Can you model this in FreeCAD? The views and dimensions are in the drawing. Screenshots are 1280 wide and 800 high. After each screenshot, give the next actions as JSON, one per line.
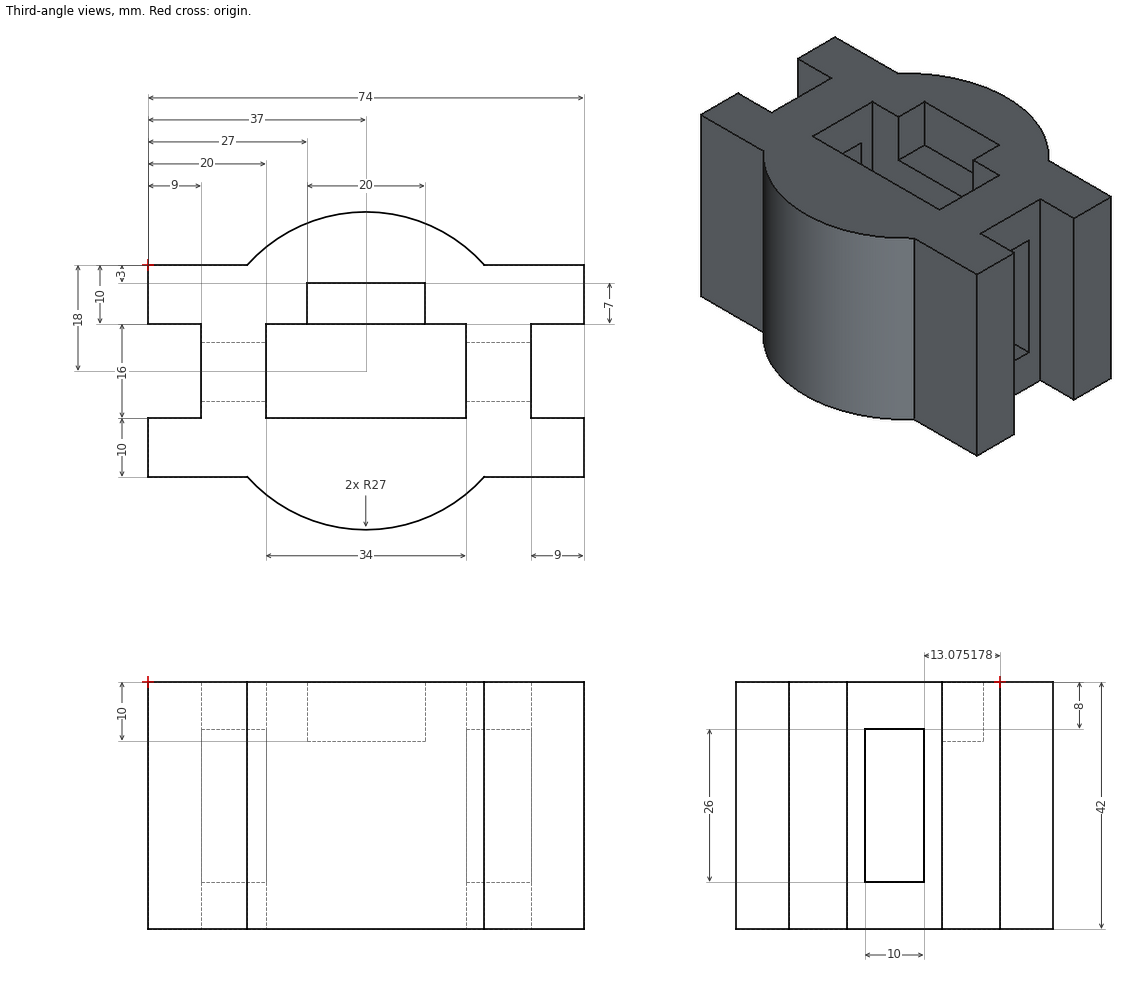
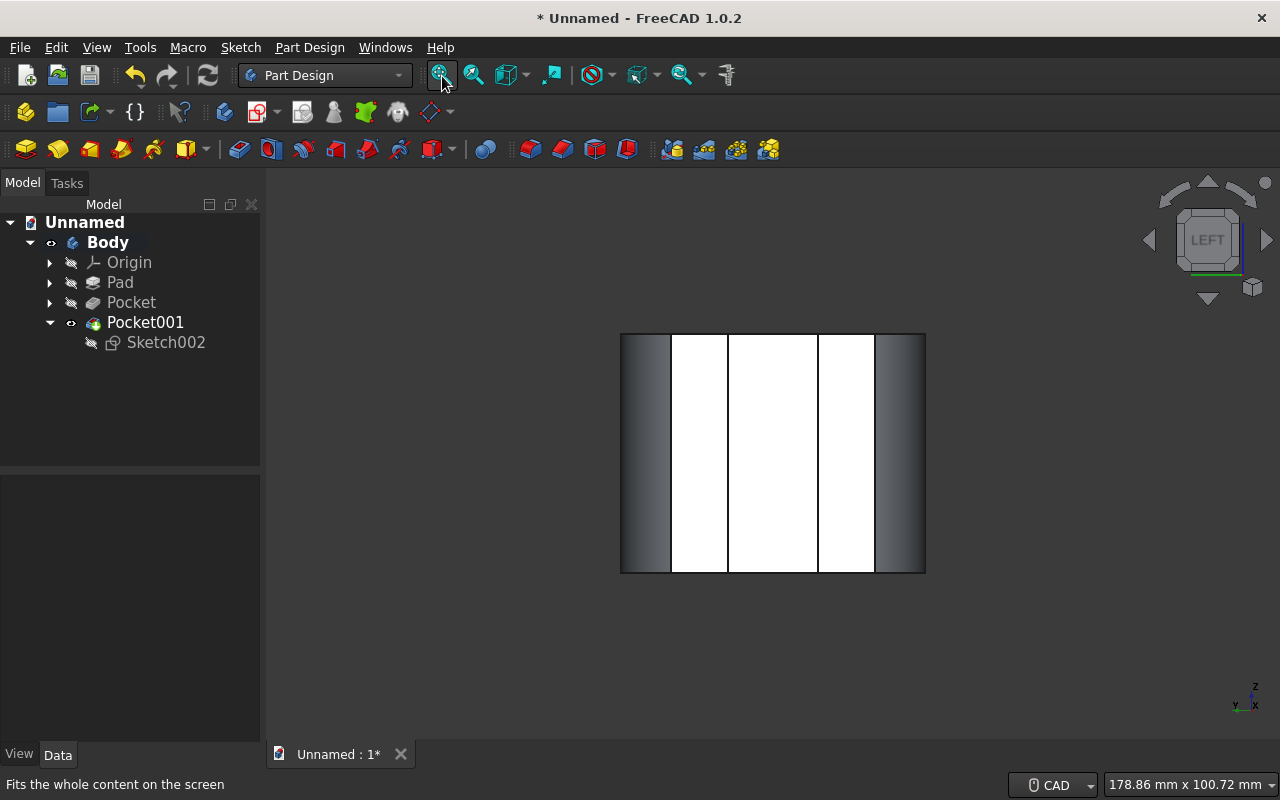
{"action": "left_click", "coordinate": [773, 384]}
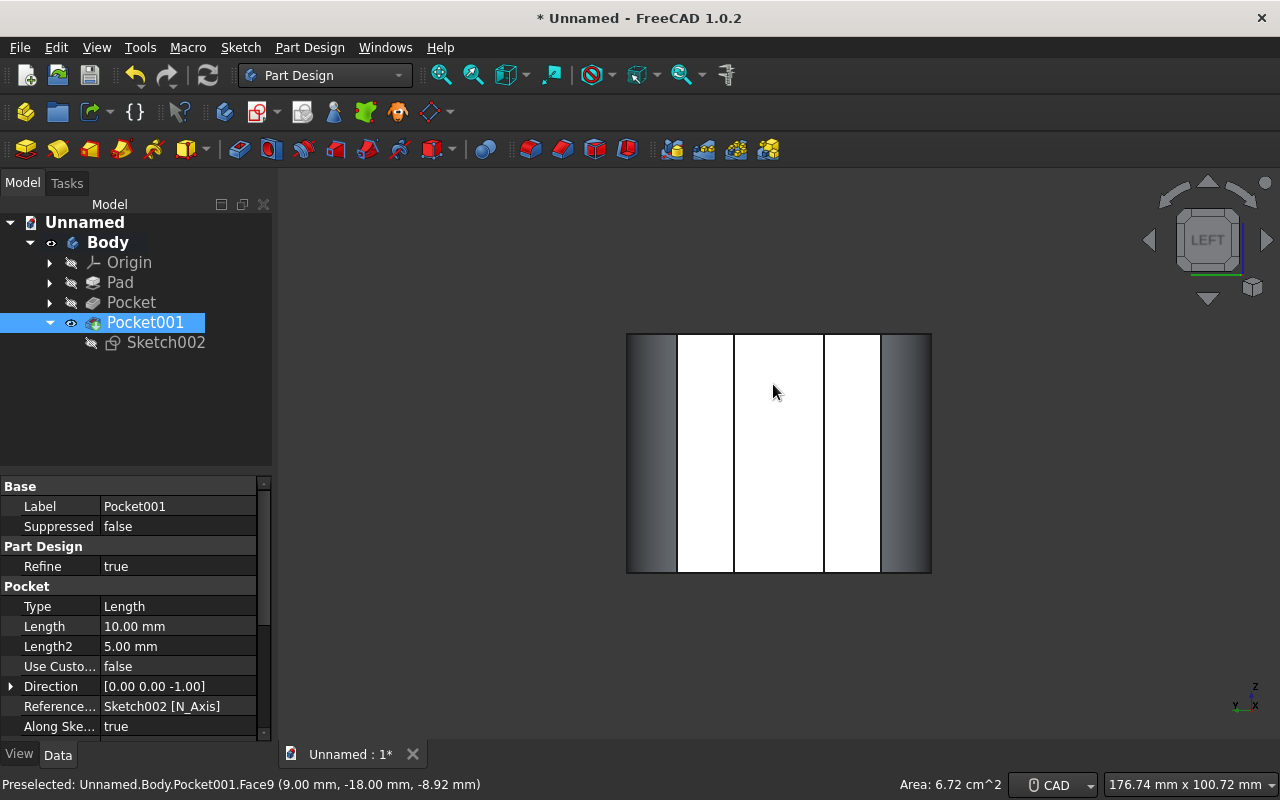
{"action": "left_click", "coordinate": [258, 112]}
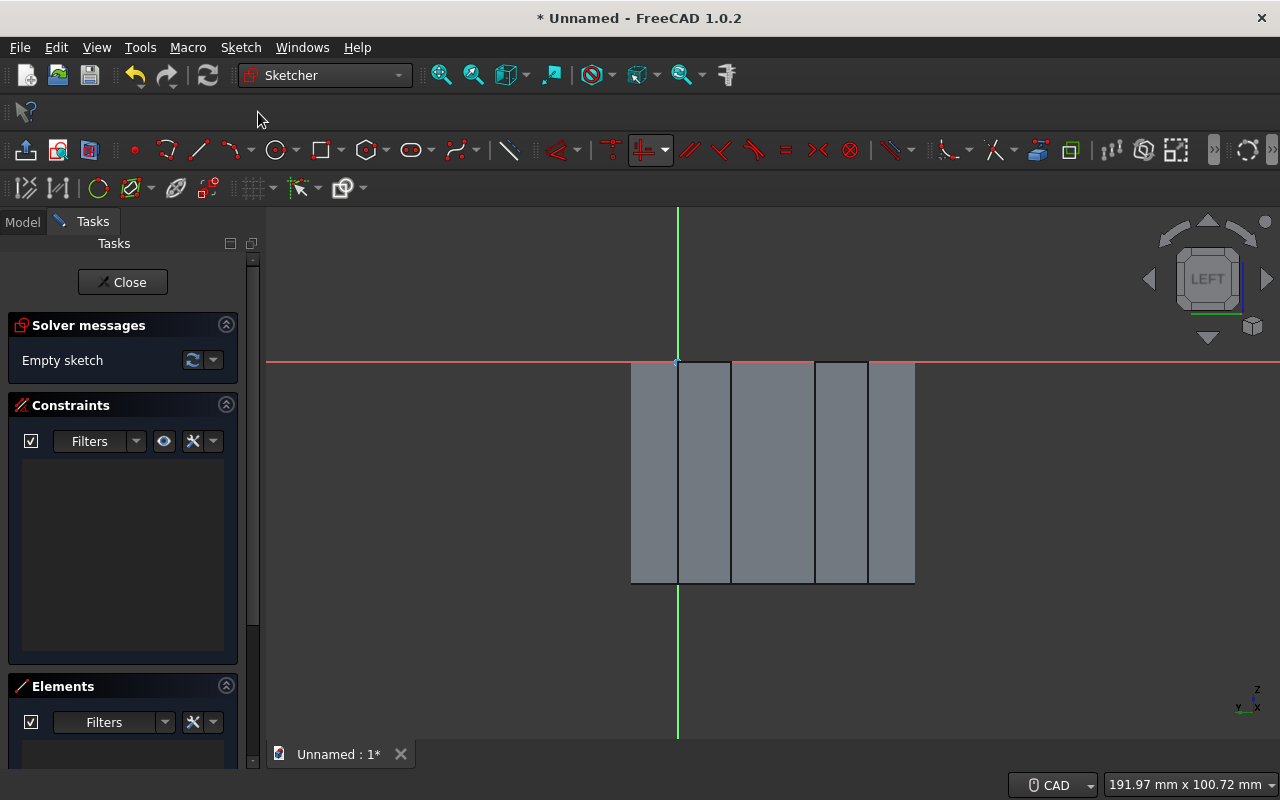
{"action": "scroll", "coordinate": [781, 426], "scroll_direction": "up", "scroll_amount": 3}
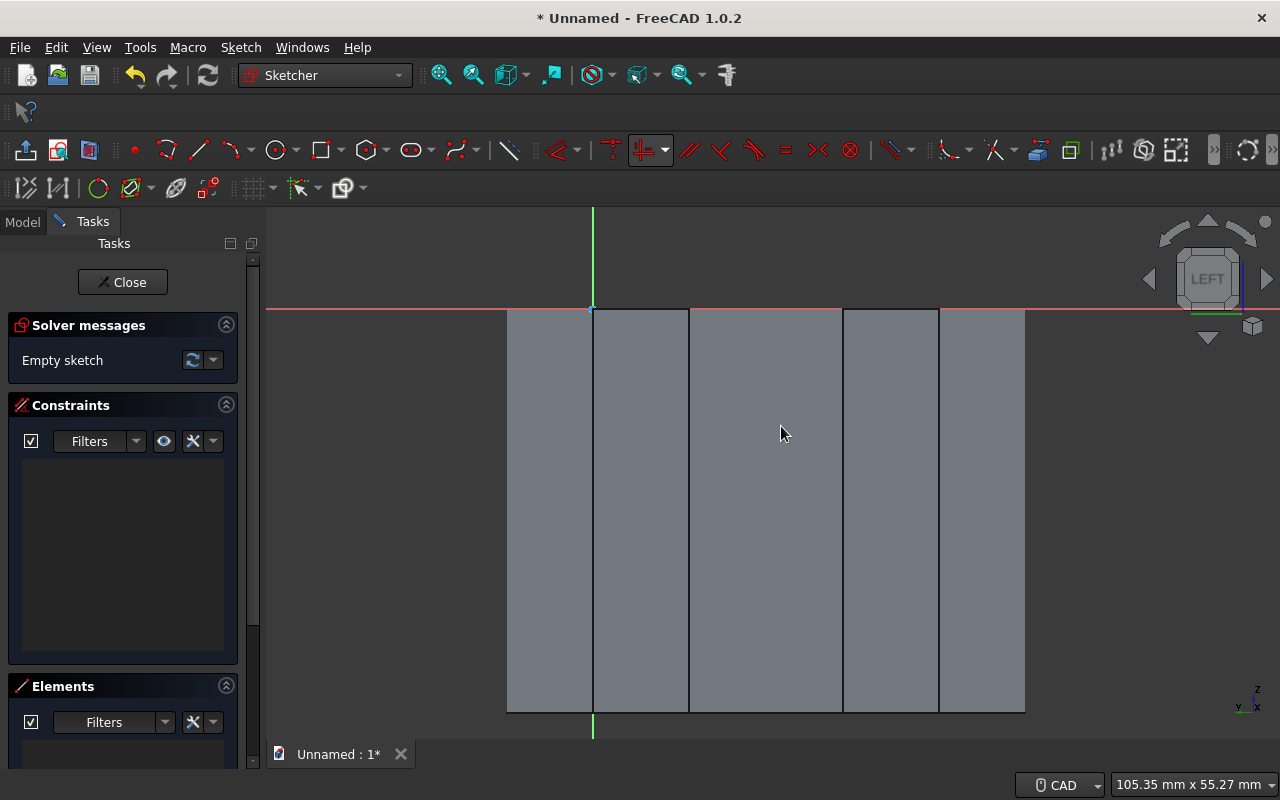
{"action": "left_click", "coordinate": [322, 150]}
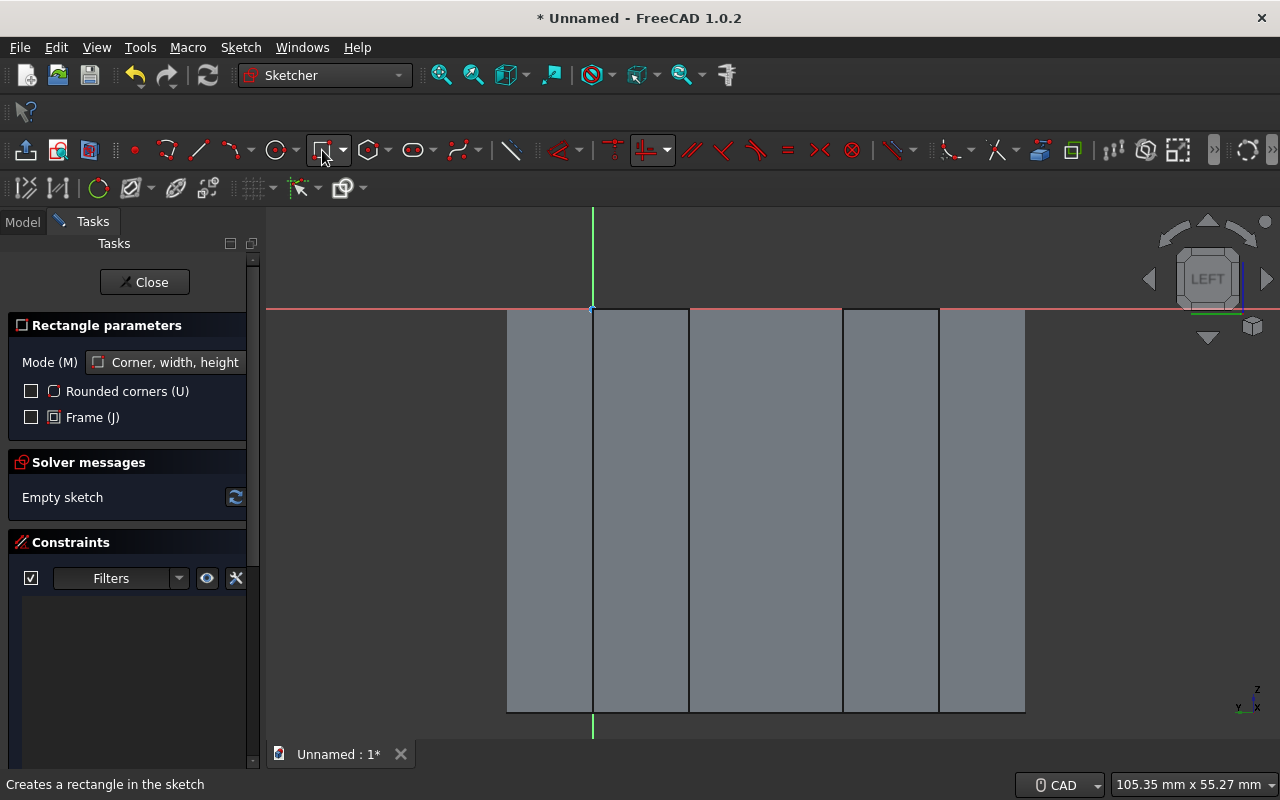
{"action": "left_click", "coordinate": [719, 386]}
{"action": "mouse_move", "coordinate": [815, 636]}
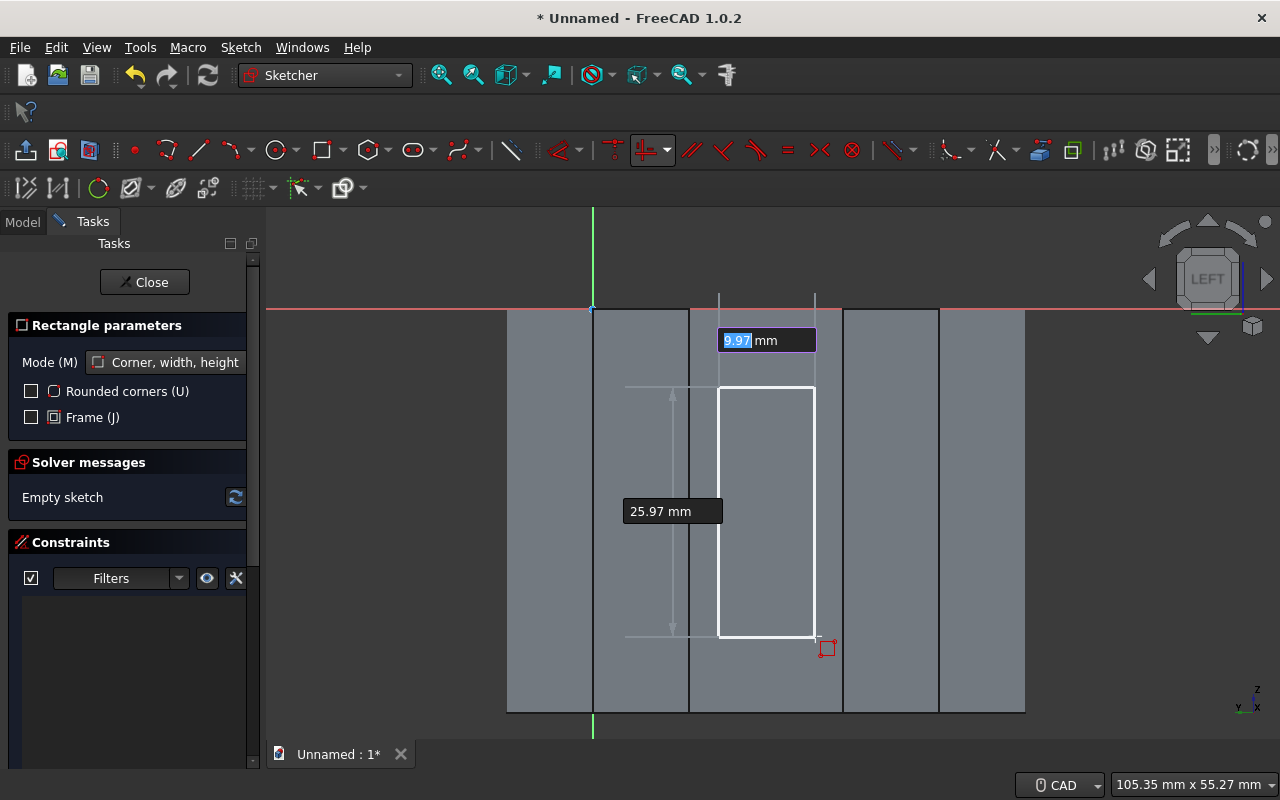
{"action": "type", "text": "10"}
{"action": "key", "text": "Tab"}
{"action": "type", "text": "26"}
{"action": "key", "text": "Return"}
{"action": "key", "text": "Escape"}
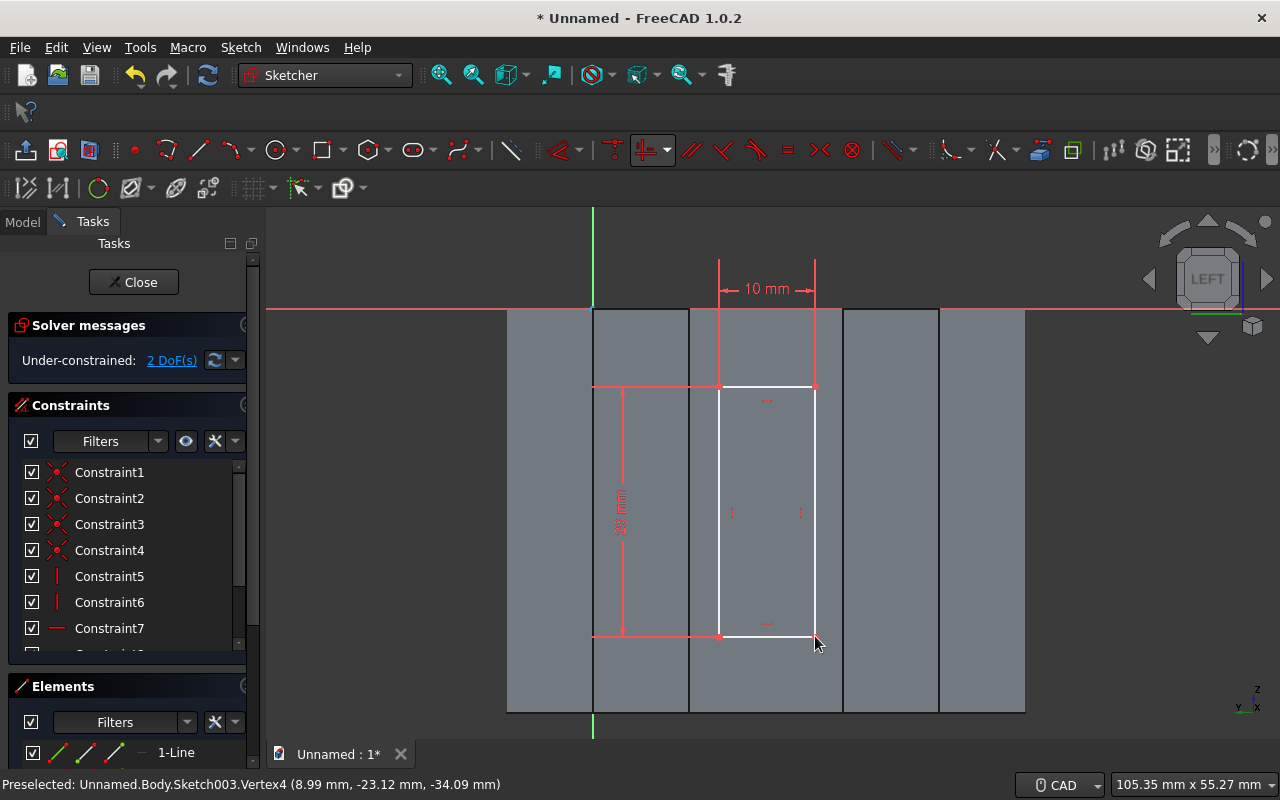
{"action": "left_click", "coordinate": [558, 150]}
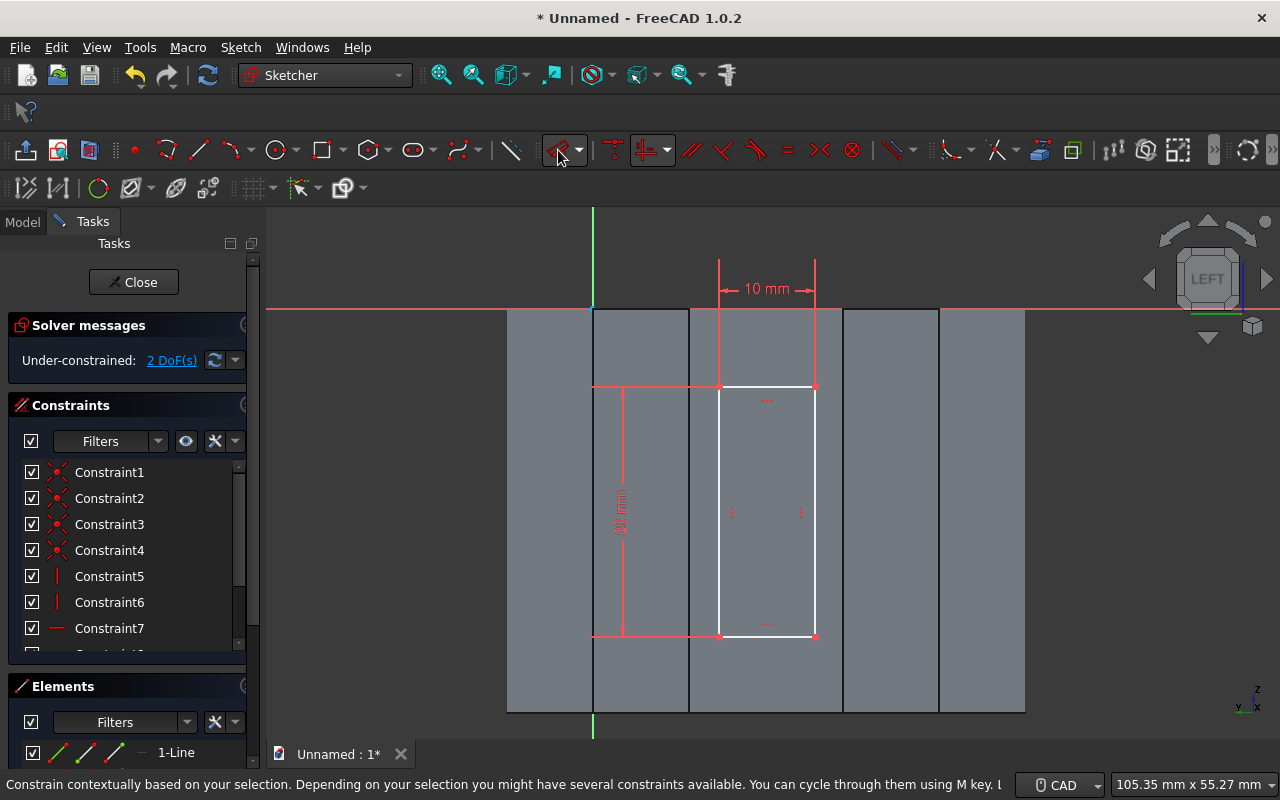
{"action": "left_click", "coordinate": [719, 387]}
{"action": "left_click", "coordinate": [559, 348]}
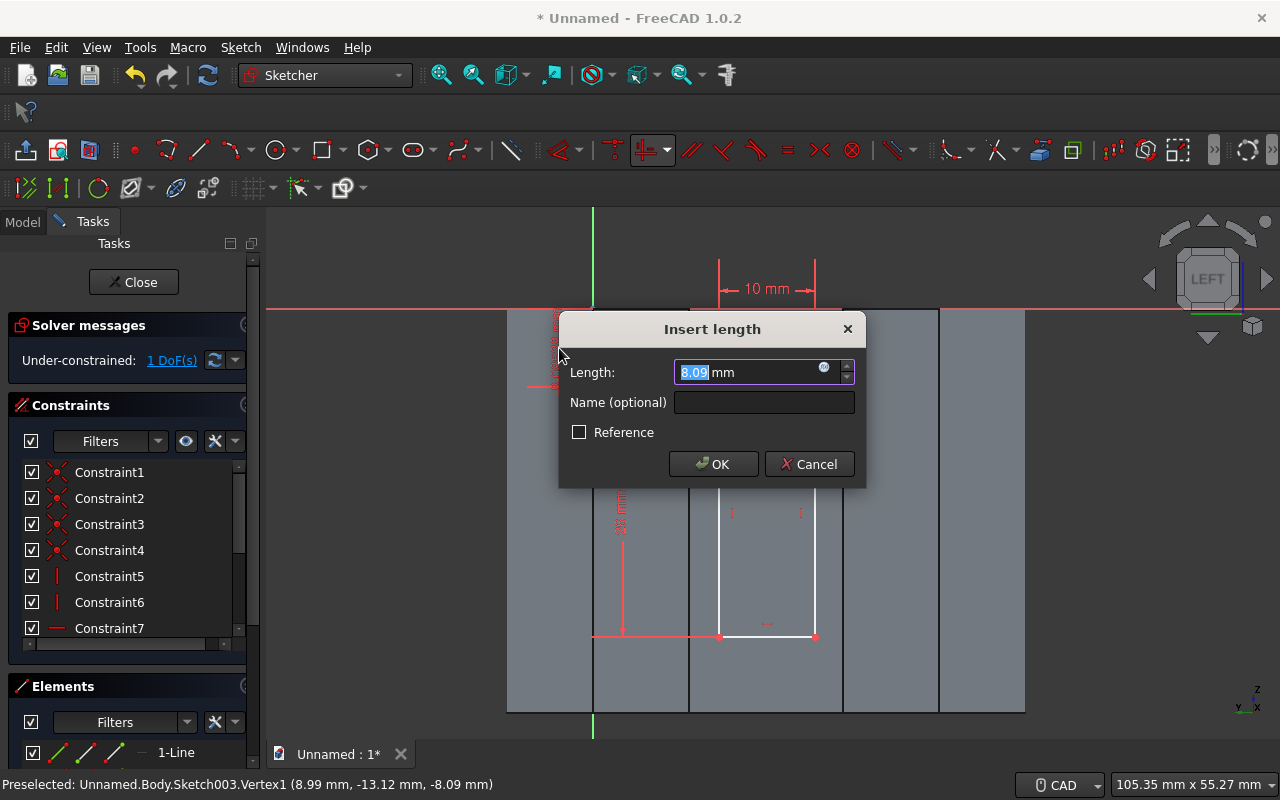
{"action": "type", "text": "8"}
{"action": "key", "text": "Return"}